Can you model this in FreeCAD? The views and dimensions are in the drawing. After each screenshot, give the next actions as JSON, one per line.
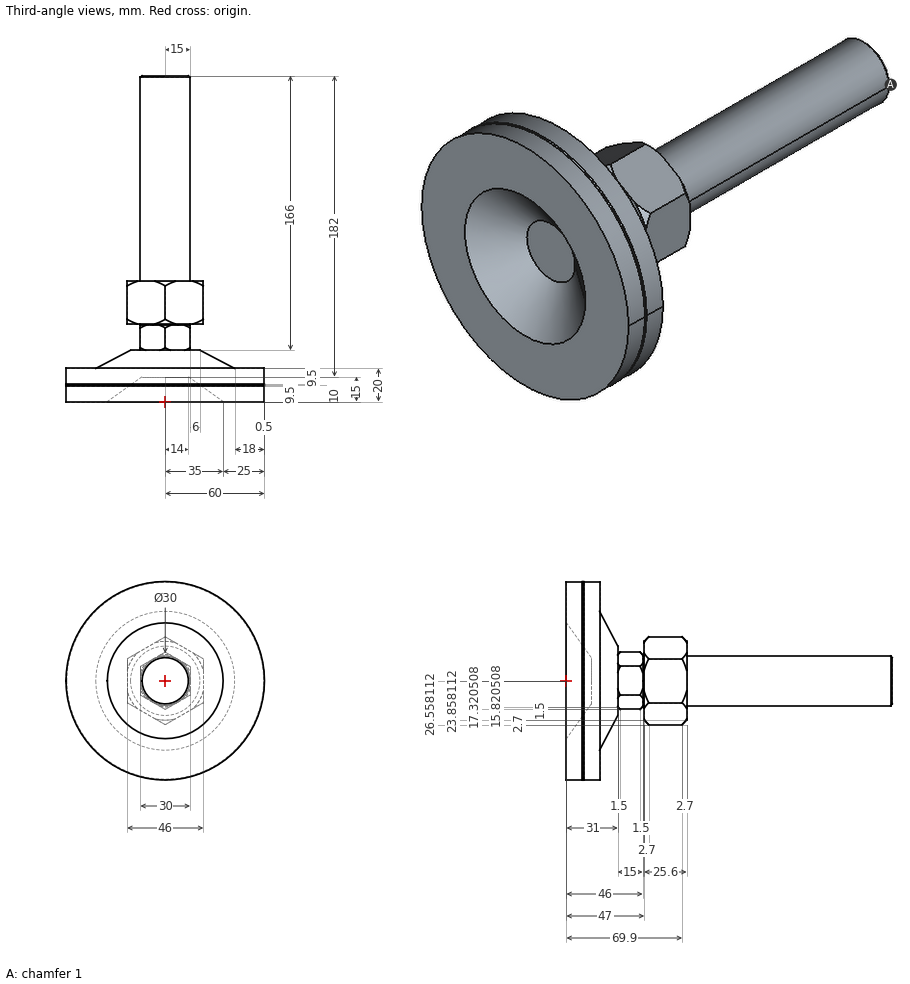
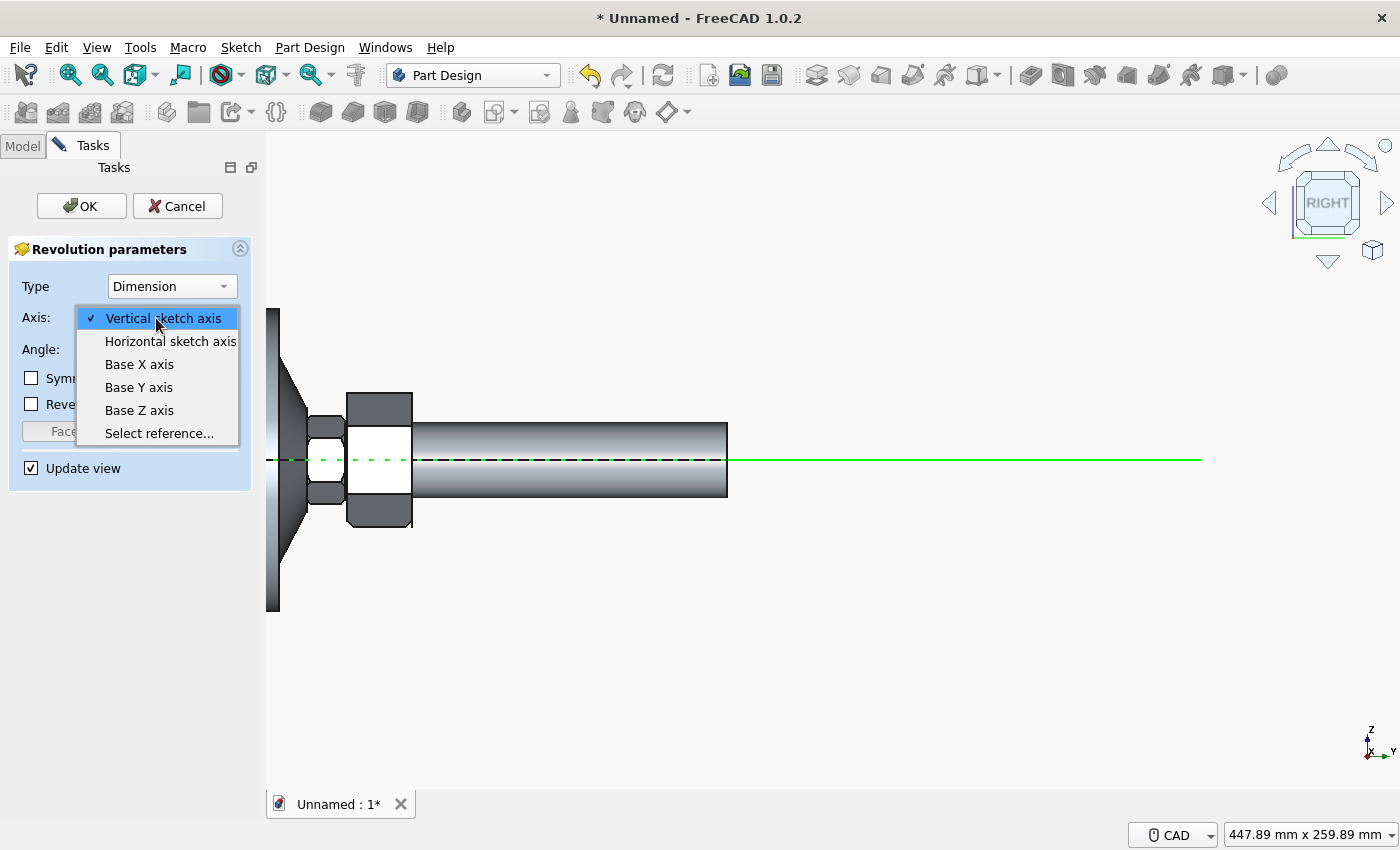
{"action": "left_click", "coordinate": [156, 342]}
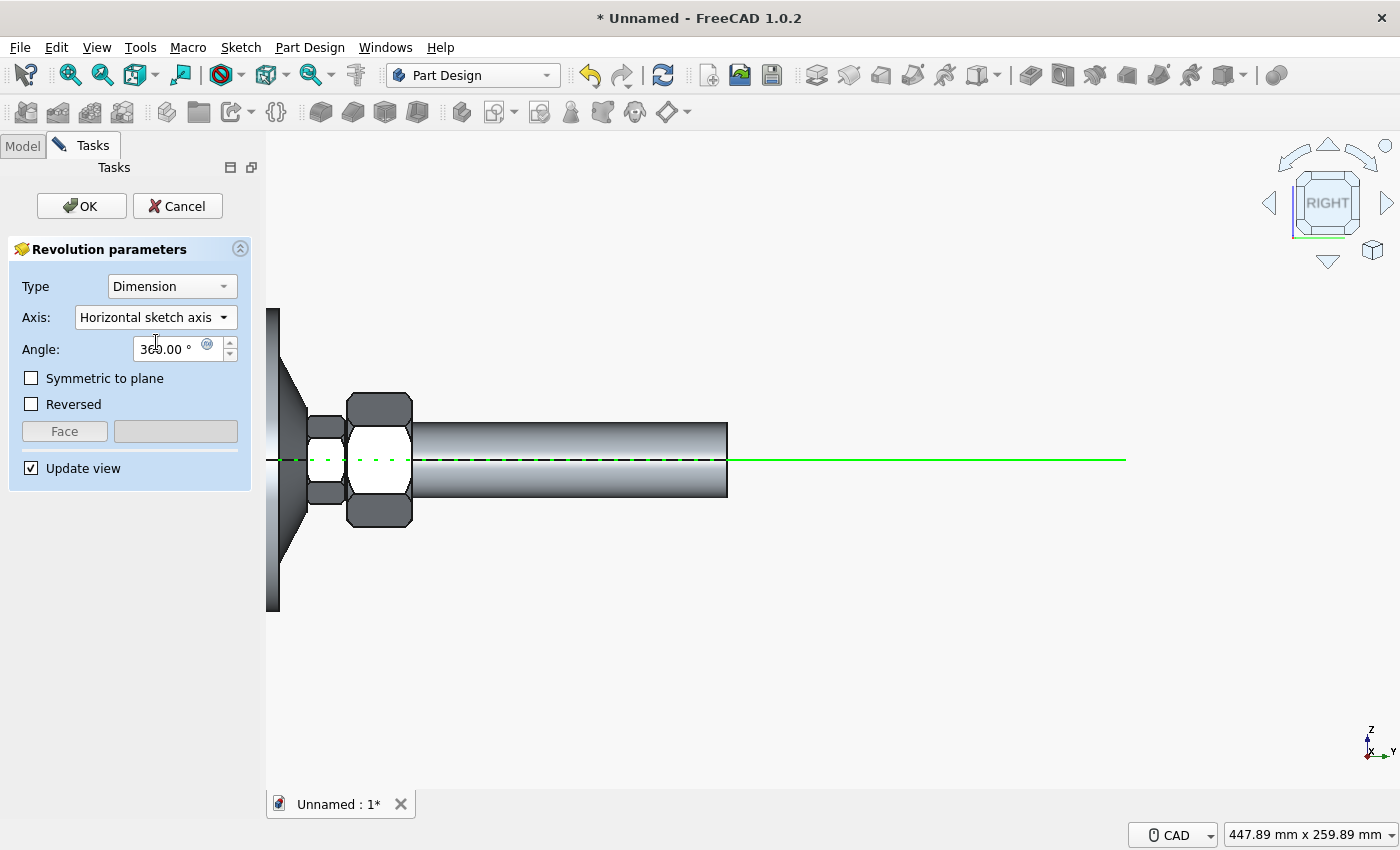
{"action": "left_click", "coordinate": [82, 206]}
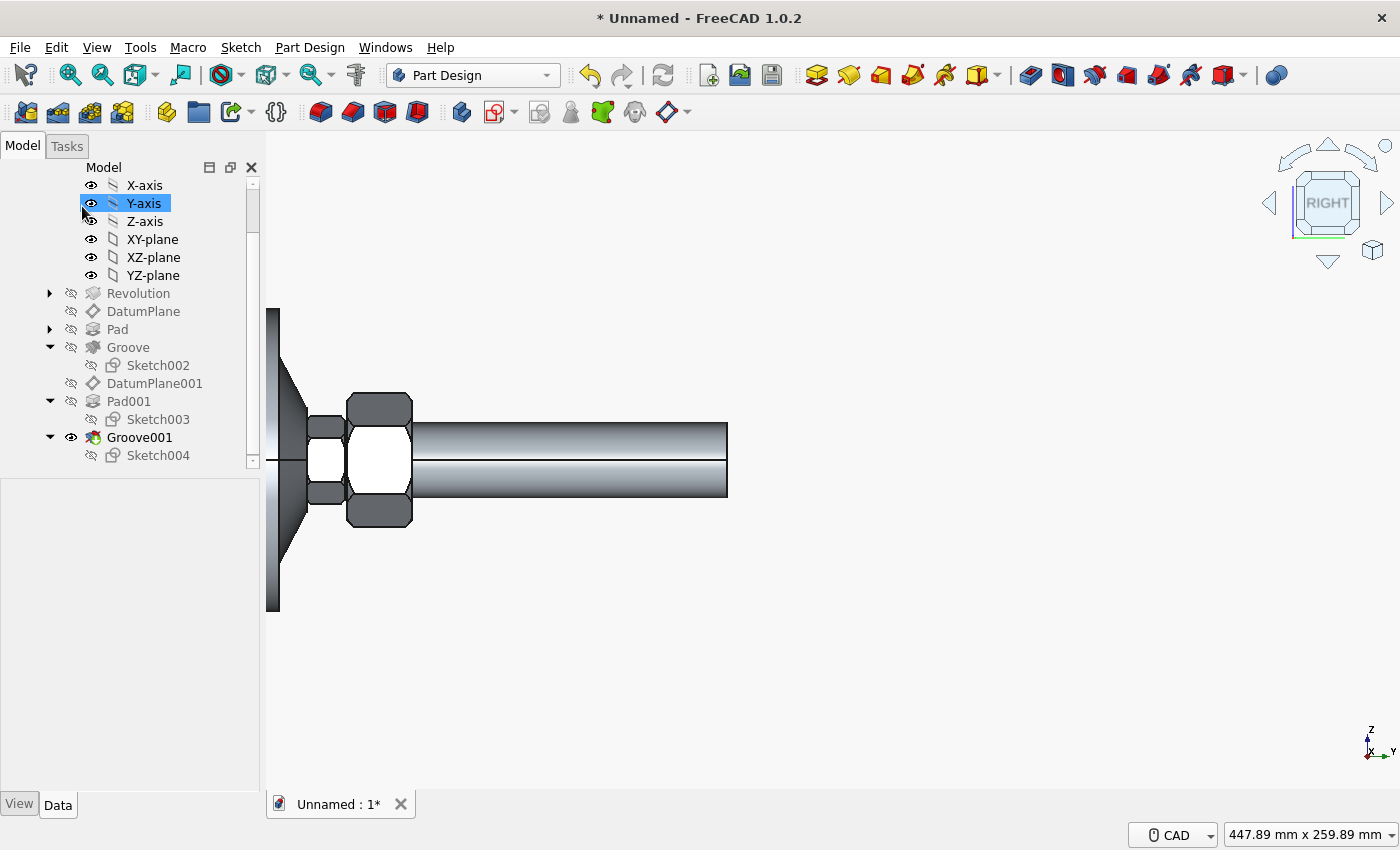
{"action": "key", "text": "v f"}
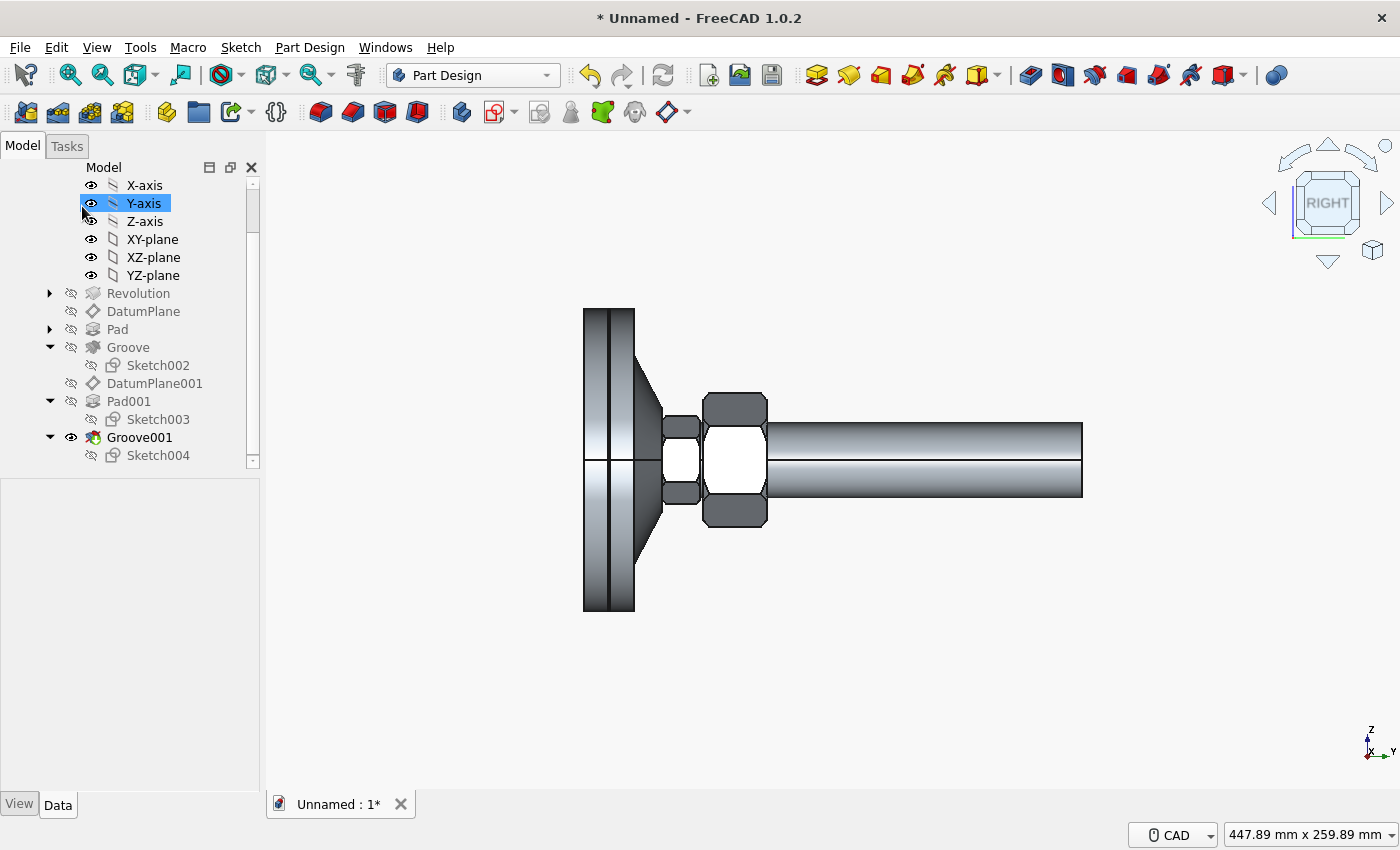
{"action": "left_click", "coordinate": [1082, 437]}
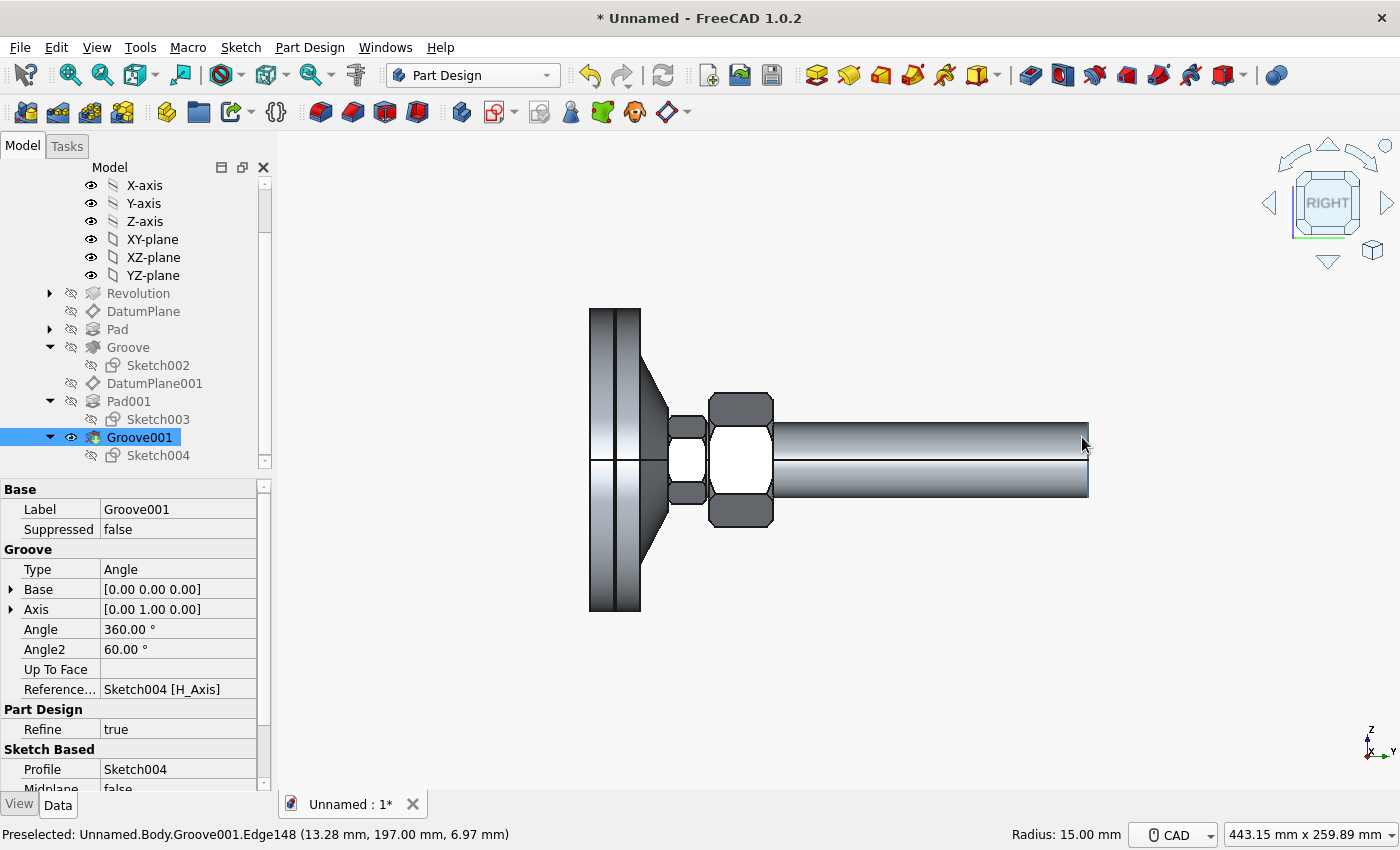
{"action": "left_click", "coordinate": [354, 112]}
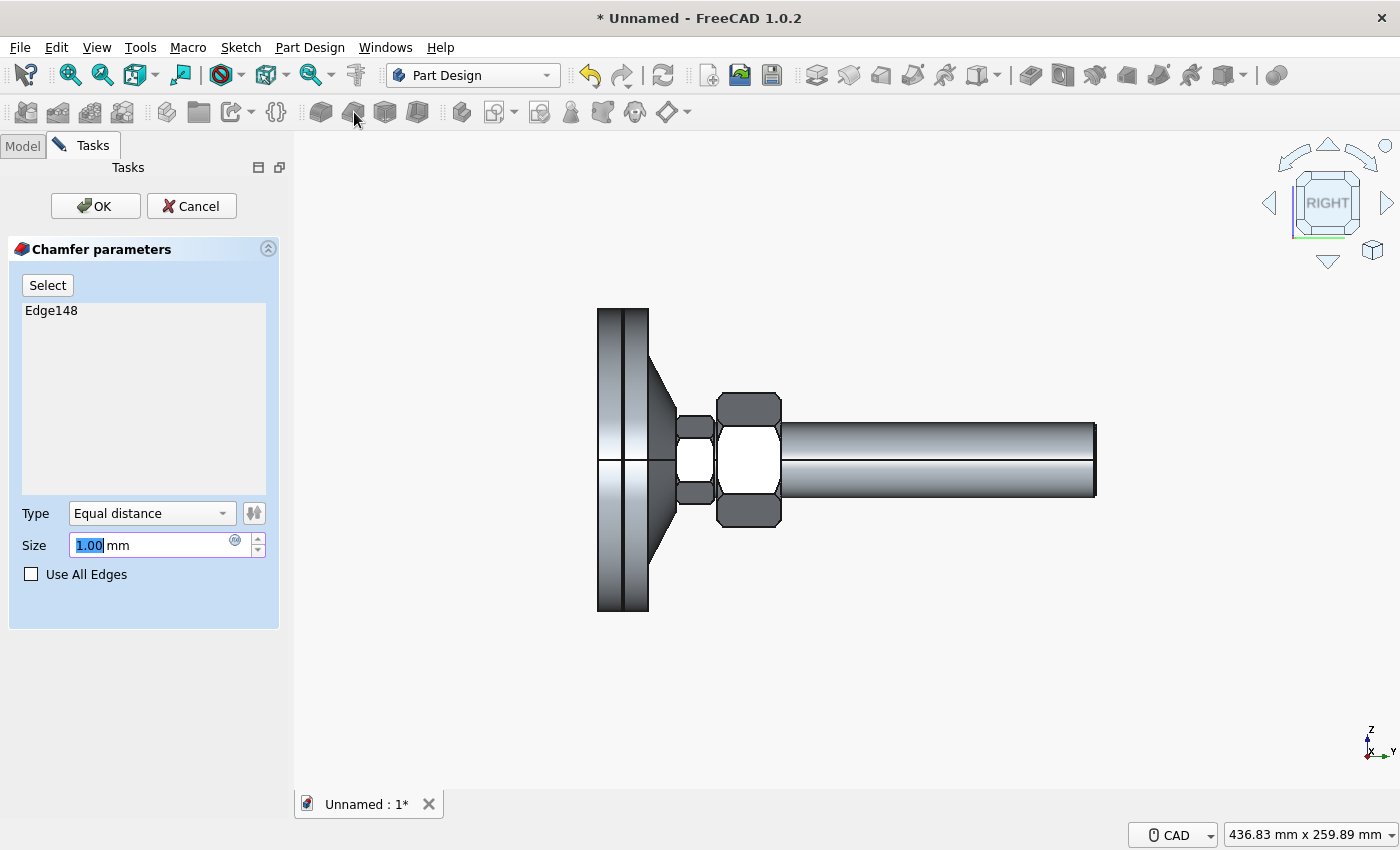
{"action": "type", "text": "1"}
{"action": "key", "text": "Tab"}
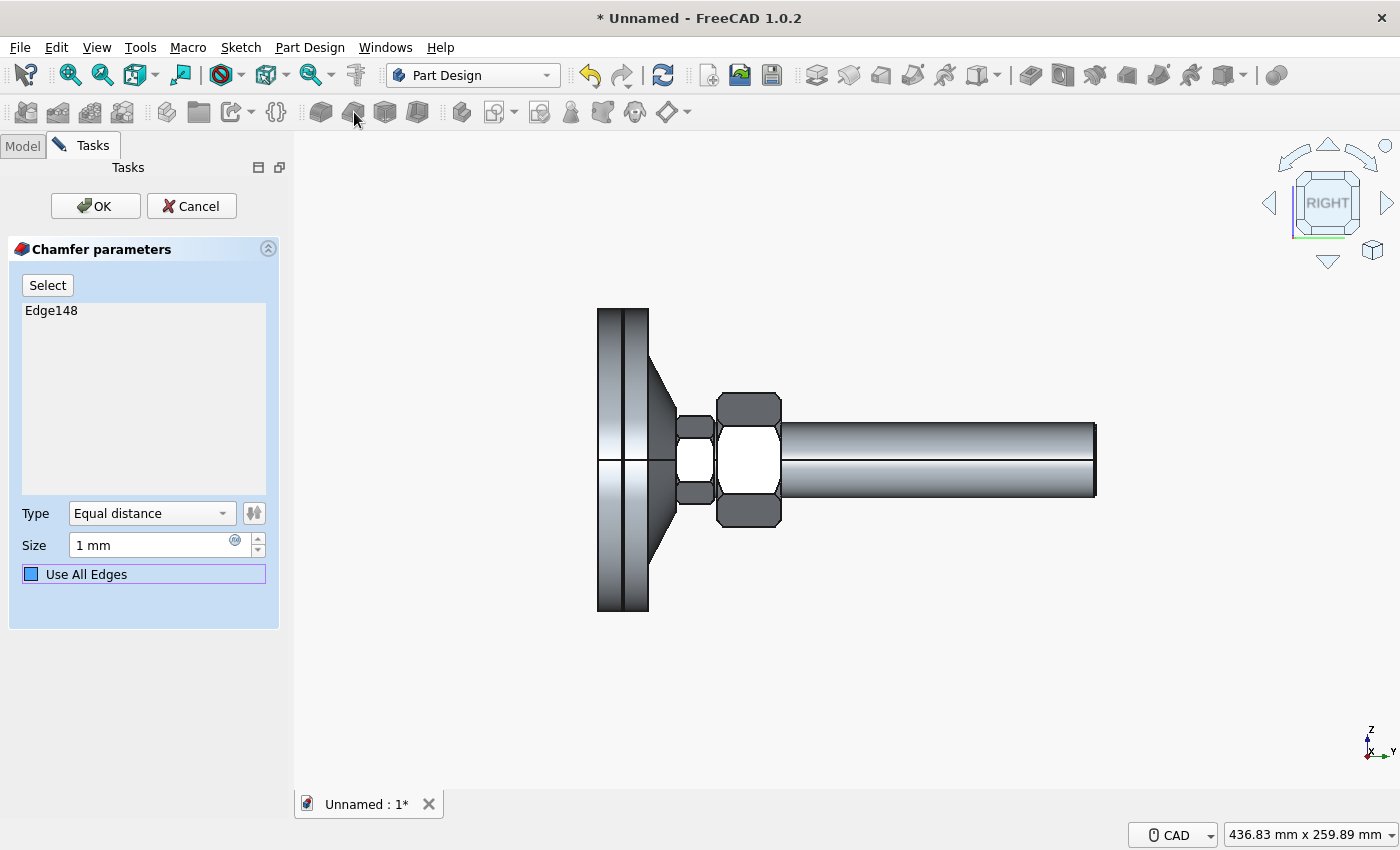
{"action": "left_click", "coordinate": [96, 206]}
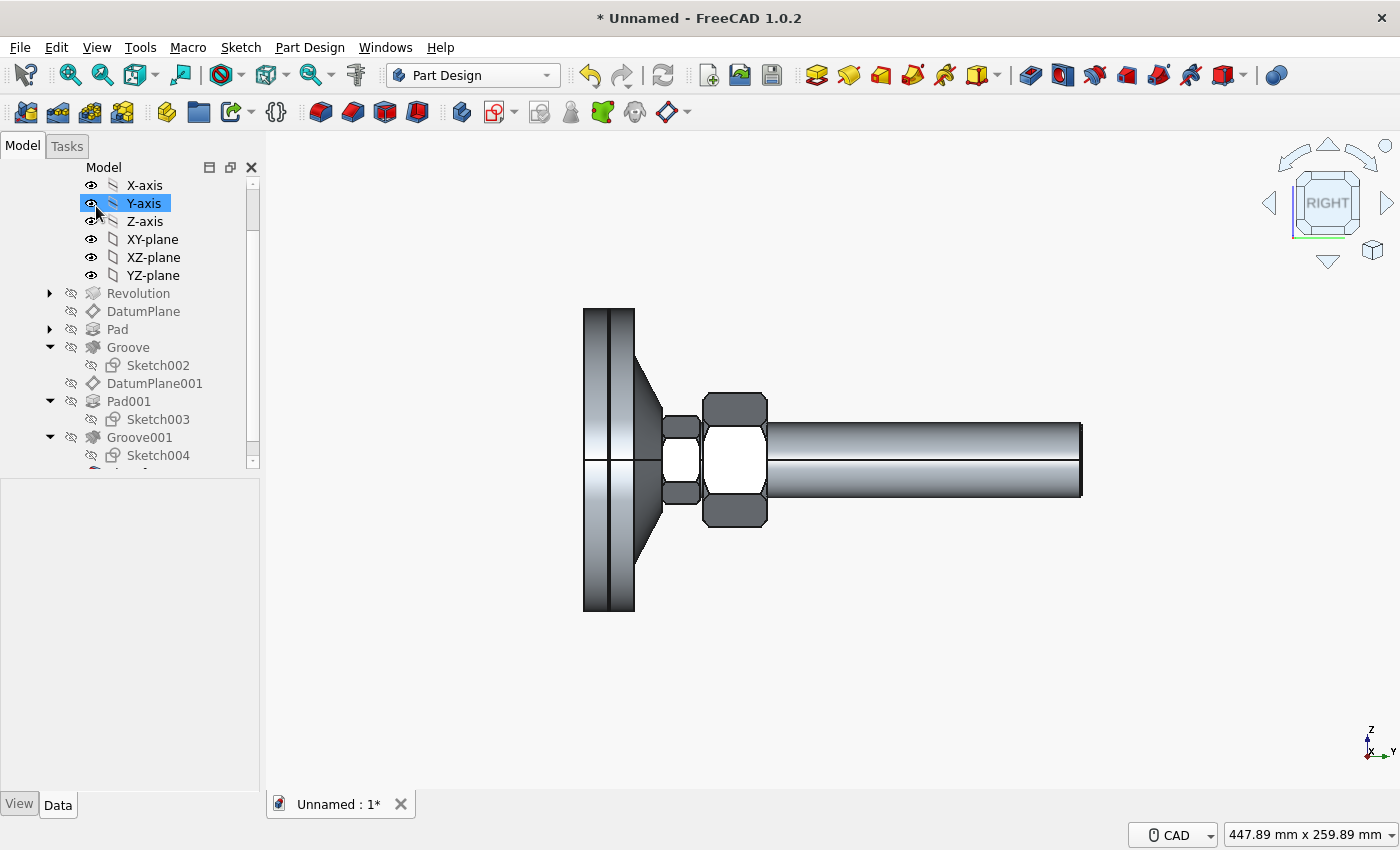
{"action": "key", "text": "0"}